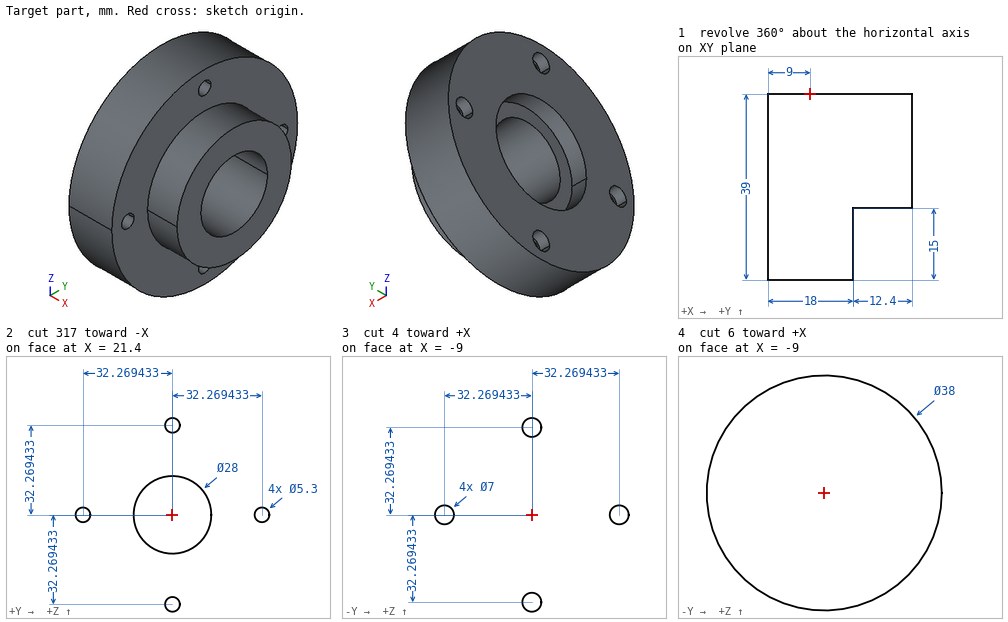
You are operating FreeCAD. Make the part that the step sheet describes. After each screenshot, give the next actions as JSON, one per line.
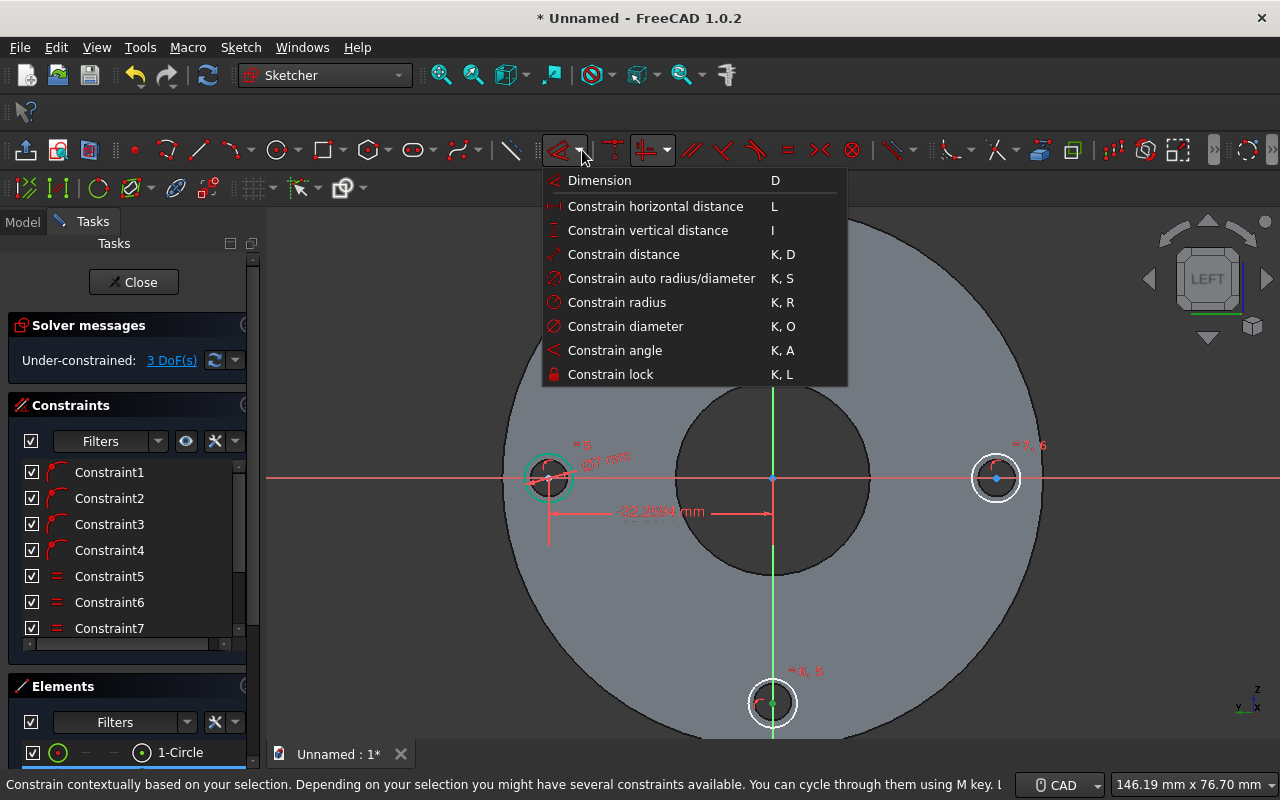
{"action": "left_click", "coordinate": [695, 230]}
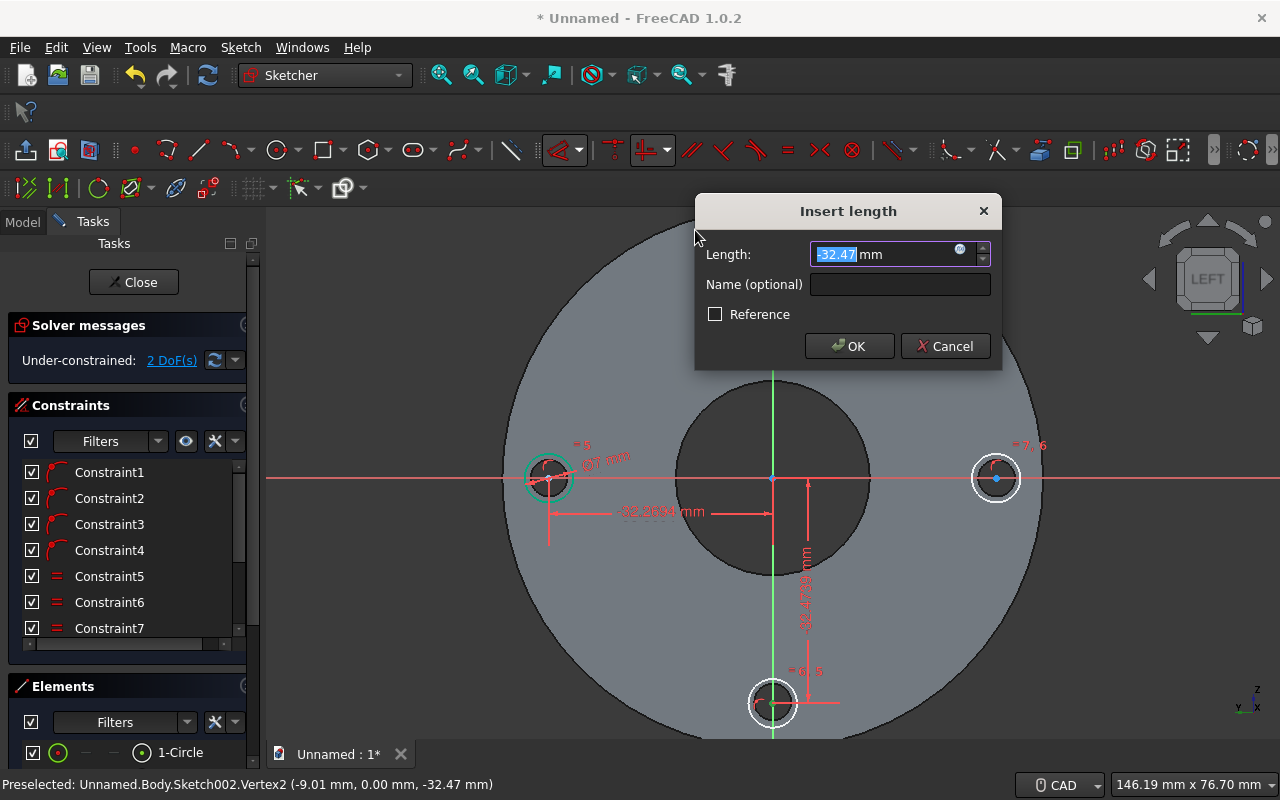
{"action": "type", "text": "-32.269433"}
{"action": "key", "text": "Return"}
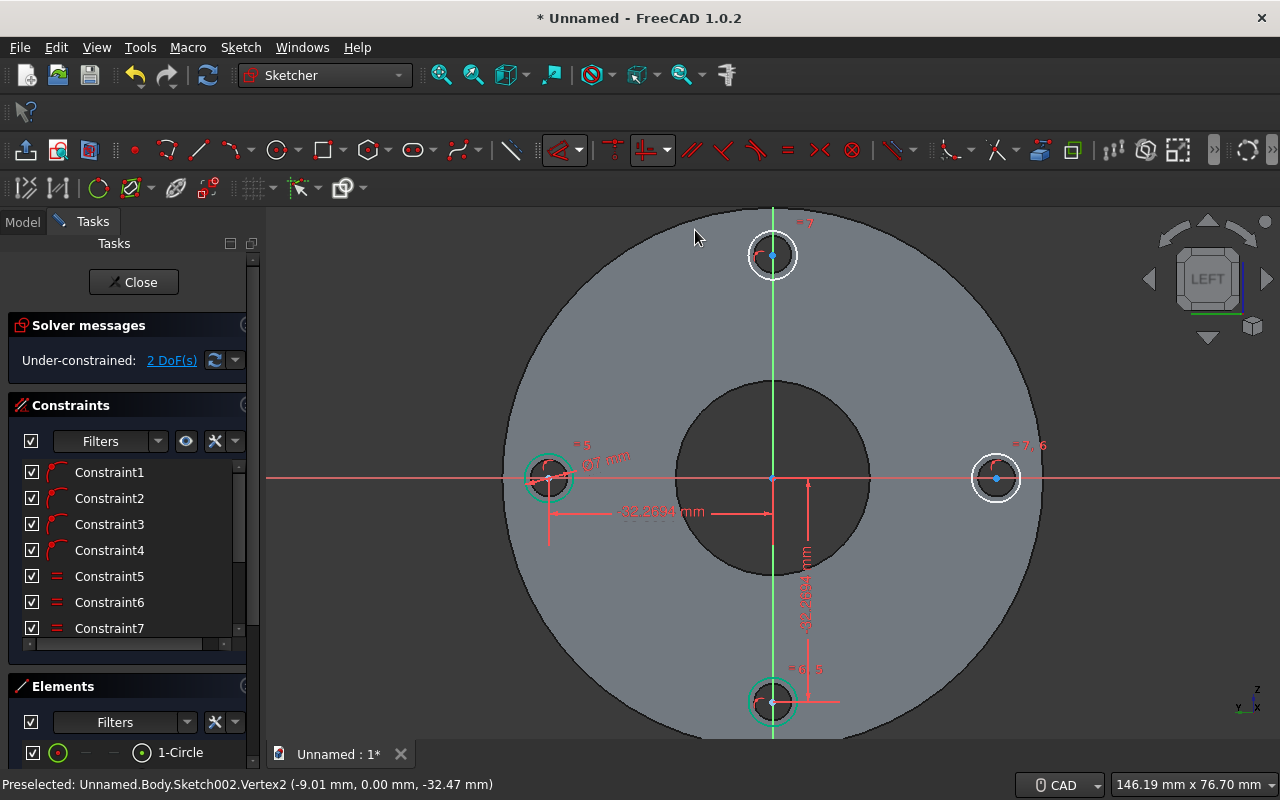
{"action": "left_click", "coordinate": [996, 478]}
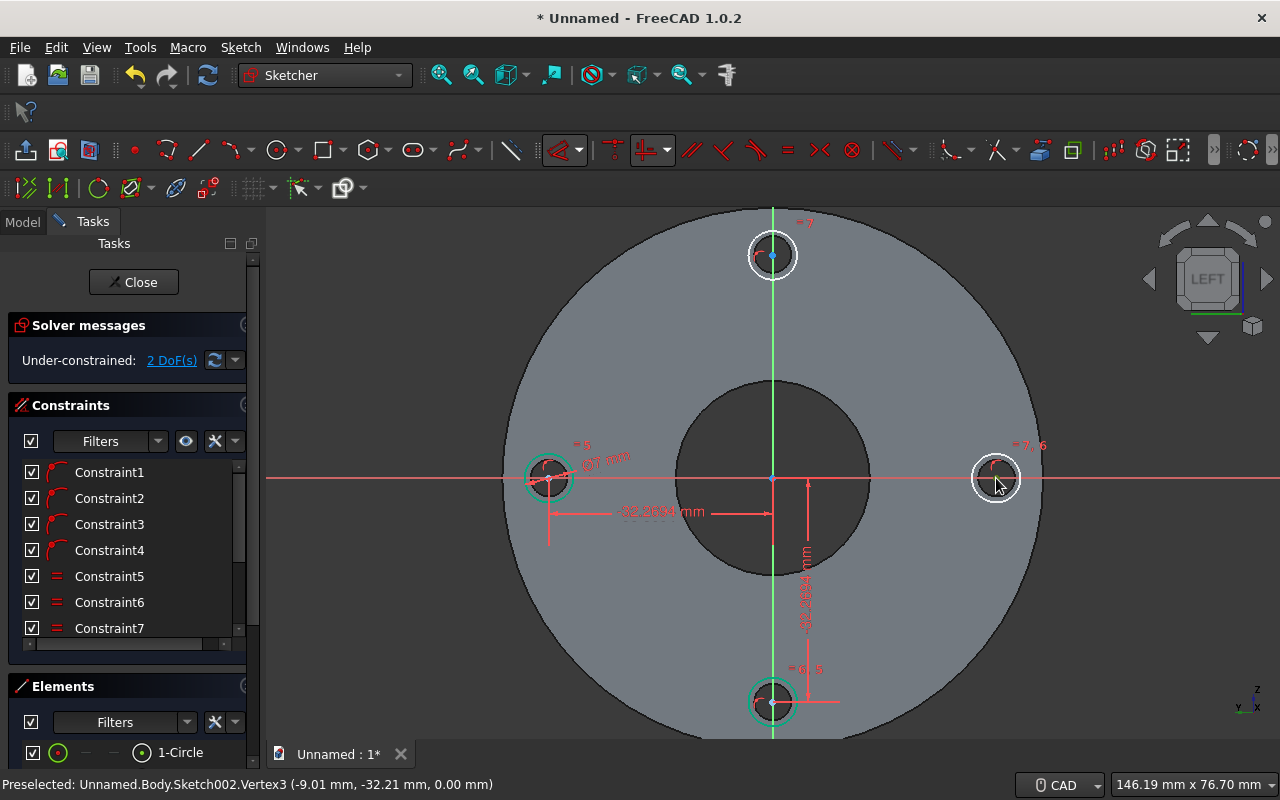
{"action": "key", "text": "l"}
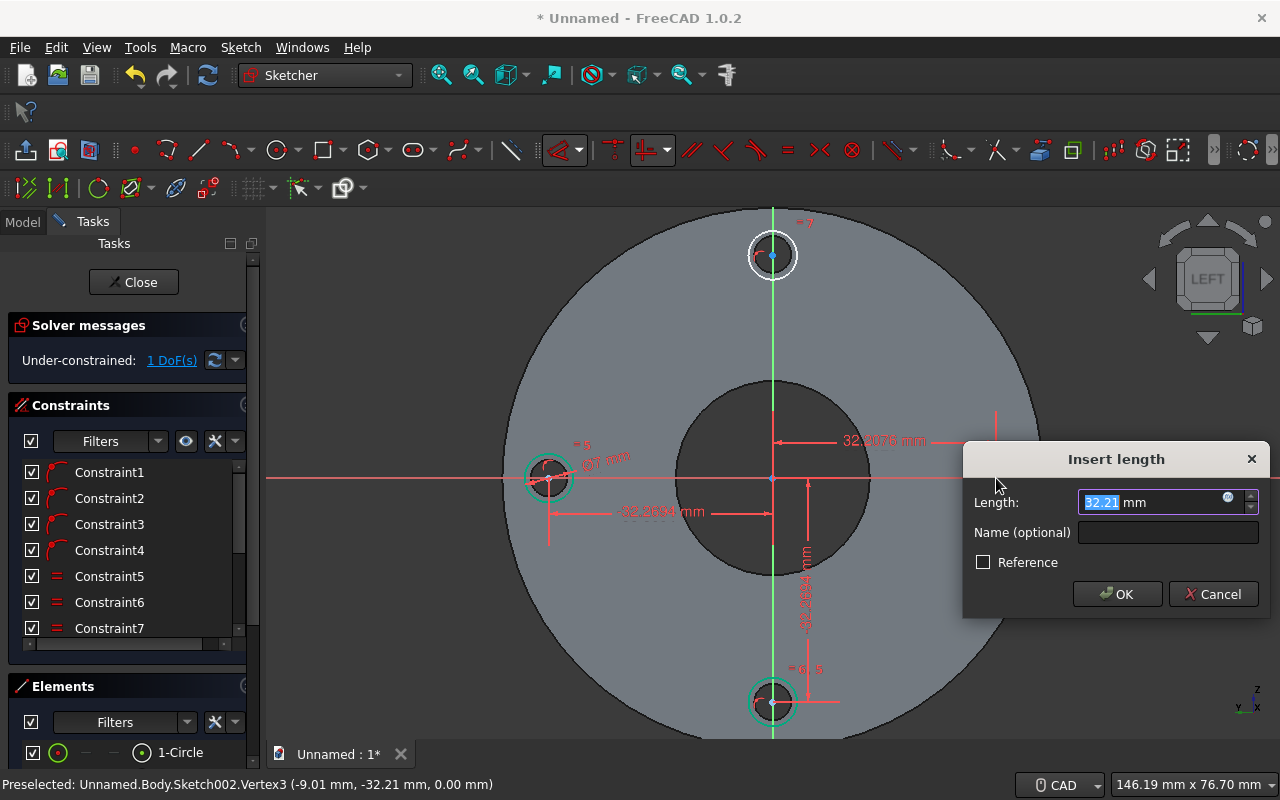
{"action": "type", "text": "32.269433"}
{"action": "key", "text": "Return"}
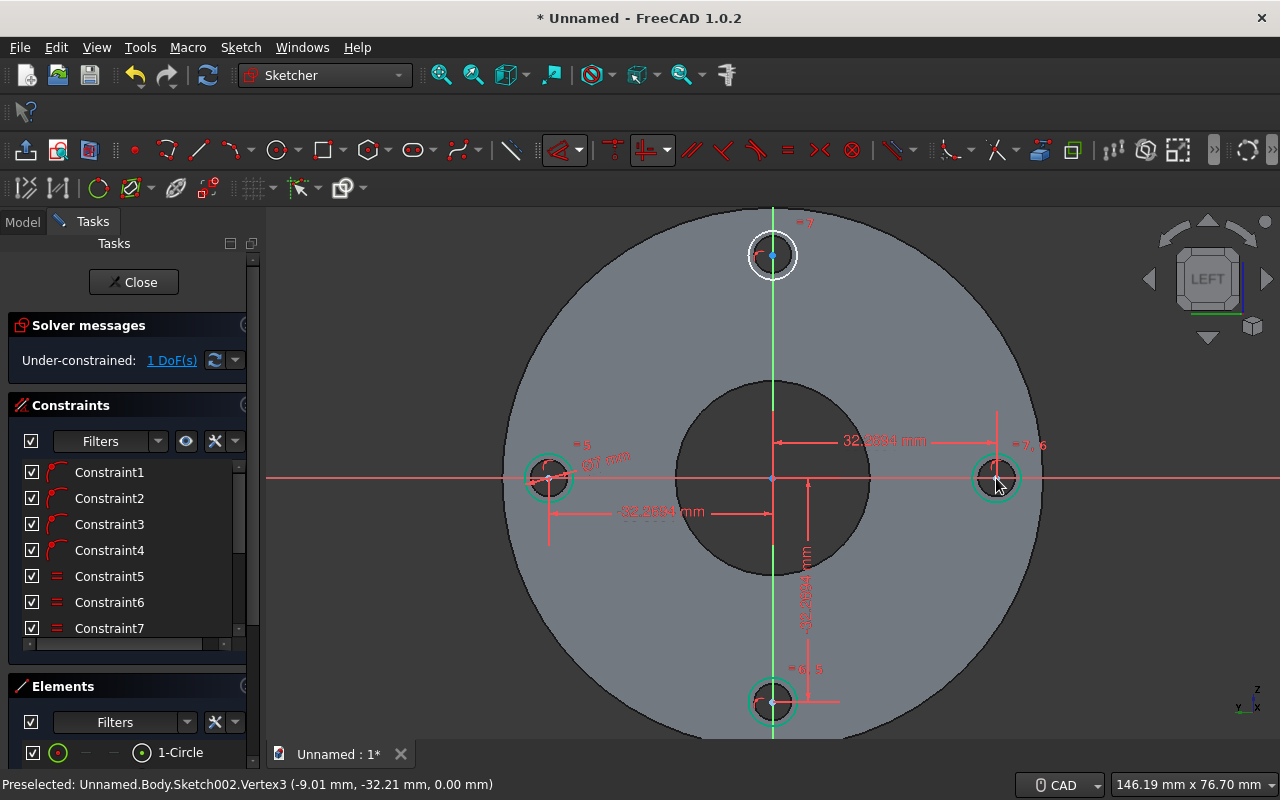
{"action": "left_click", "coordinate": [773, 255]}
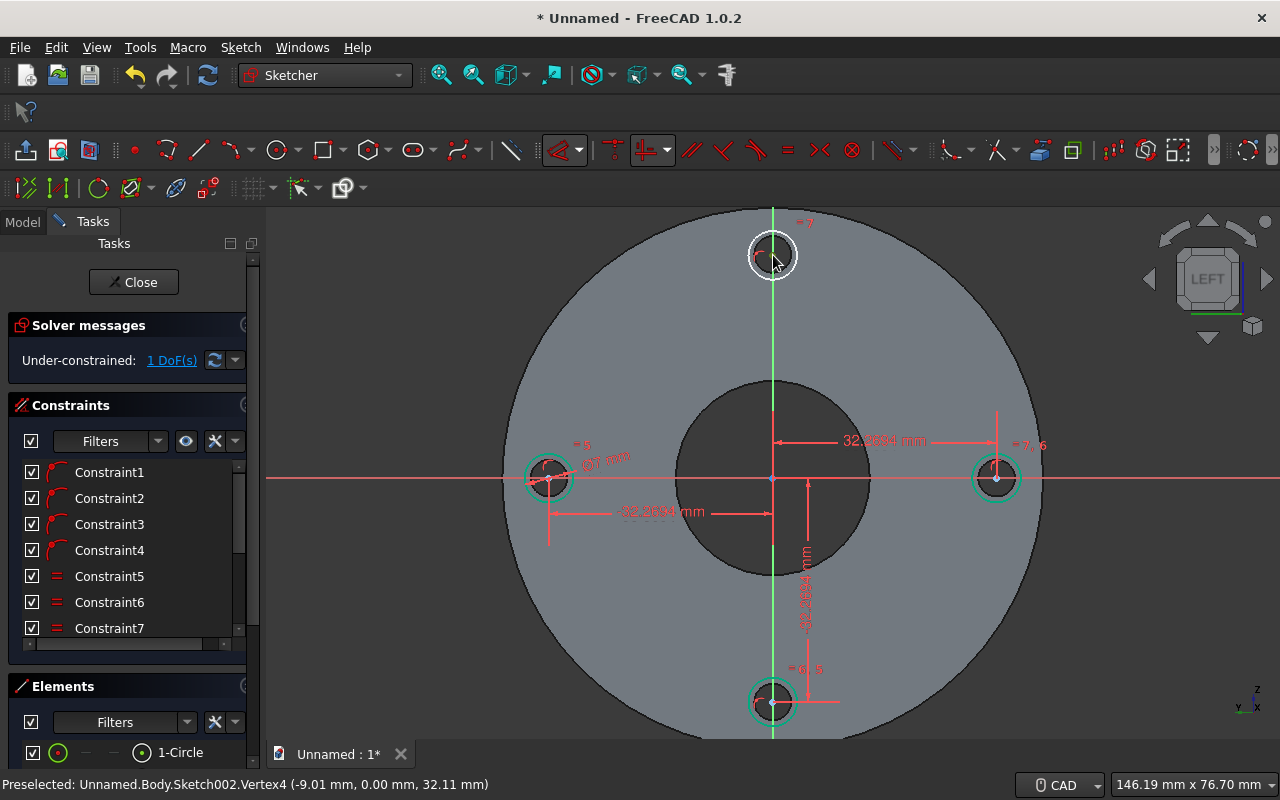
{"action": "left_click", "coordinate": [582, 150]}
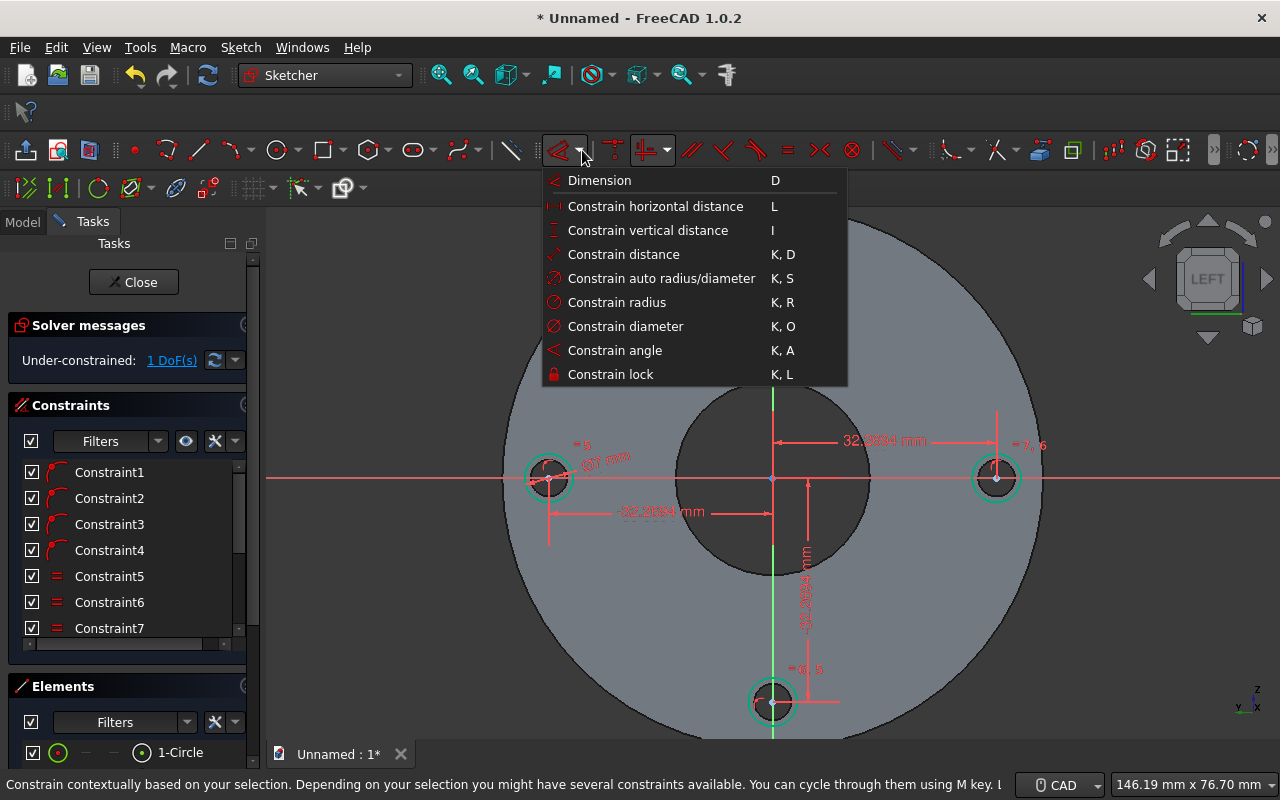
{"action": "left_click", "coordinate": [695, 230]}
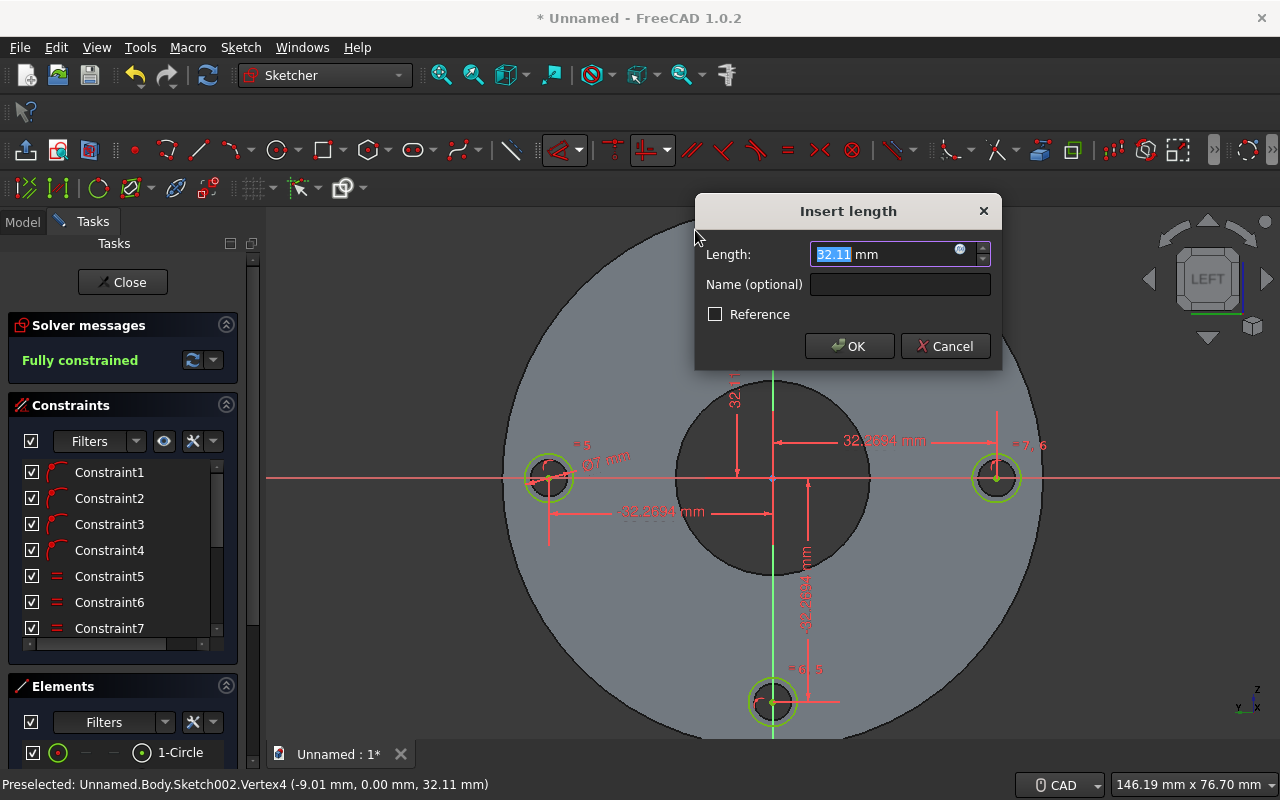
{"action": "type", "text": "32.269433"}
{"action": "key", "text": "Return"}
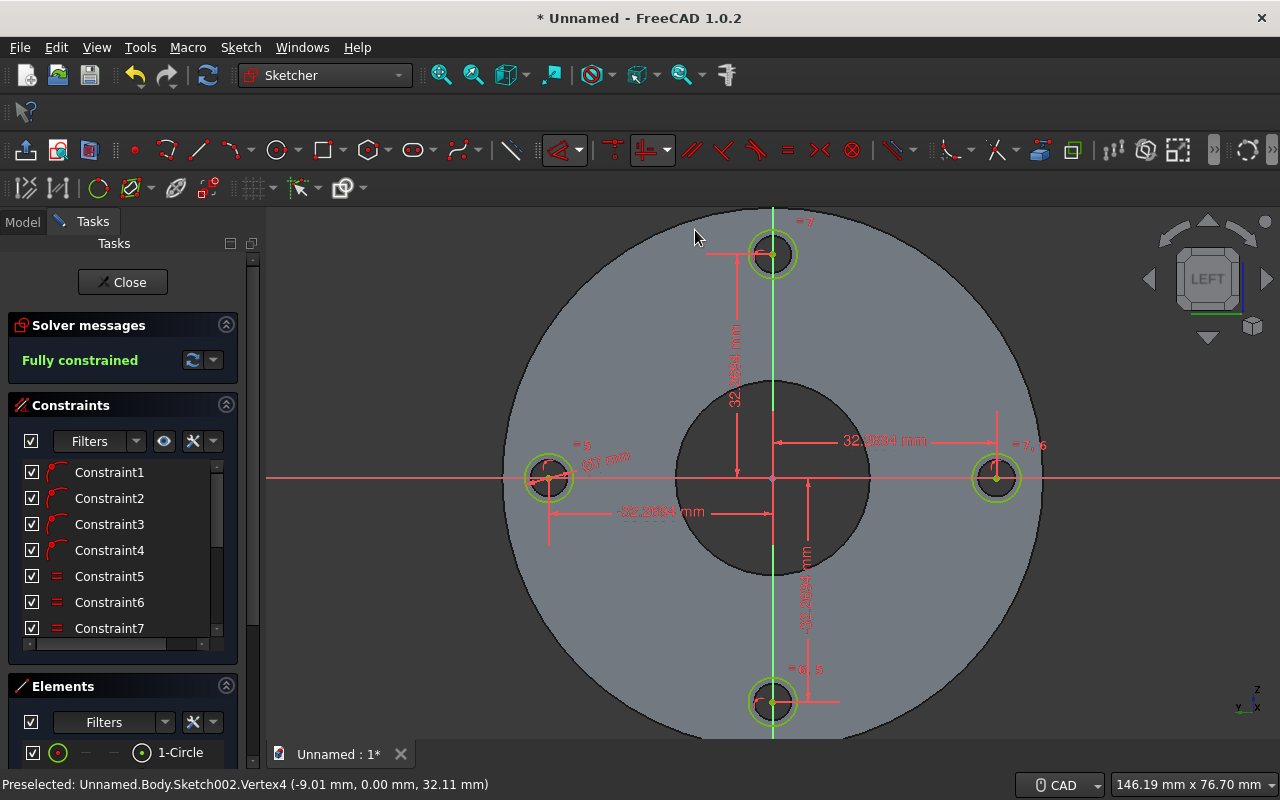
{"action": "left_click", "coordinate": [123, 282]}